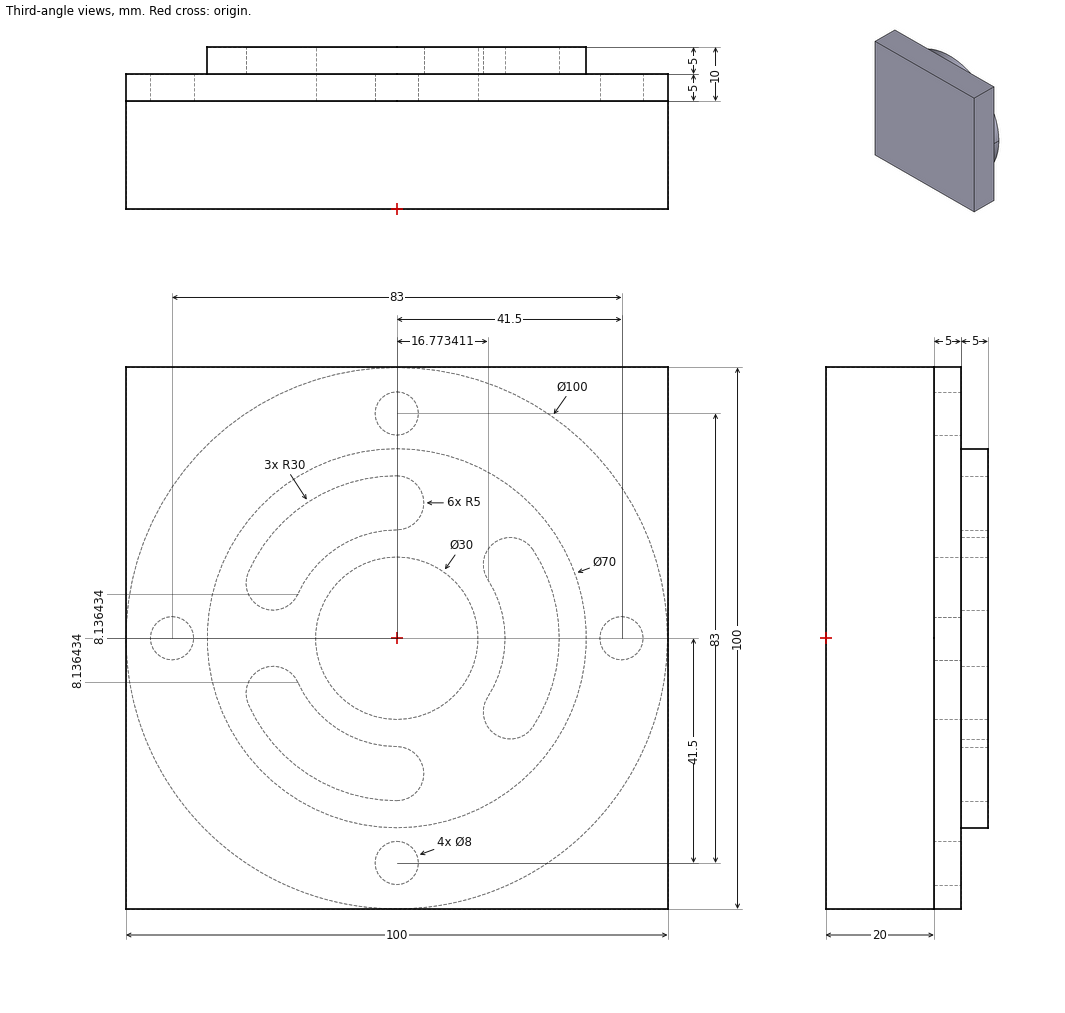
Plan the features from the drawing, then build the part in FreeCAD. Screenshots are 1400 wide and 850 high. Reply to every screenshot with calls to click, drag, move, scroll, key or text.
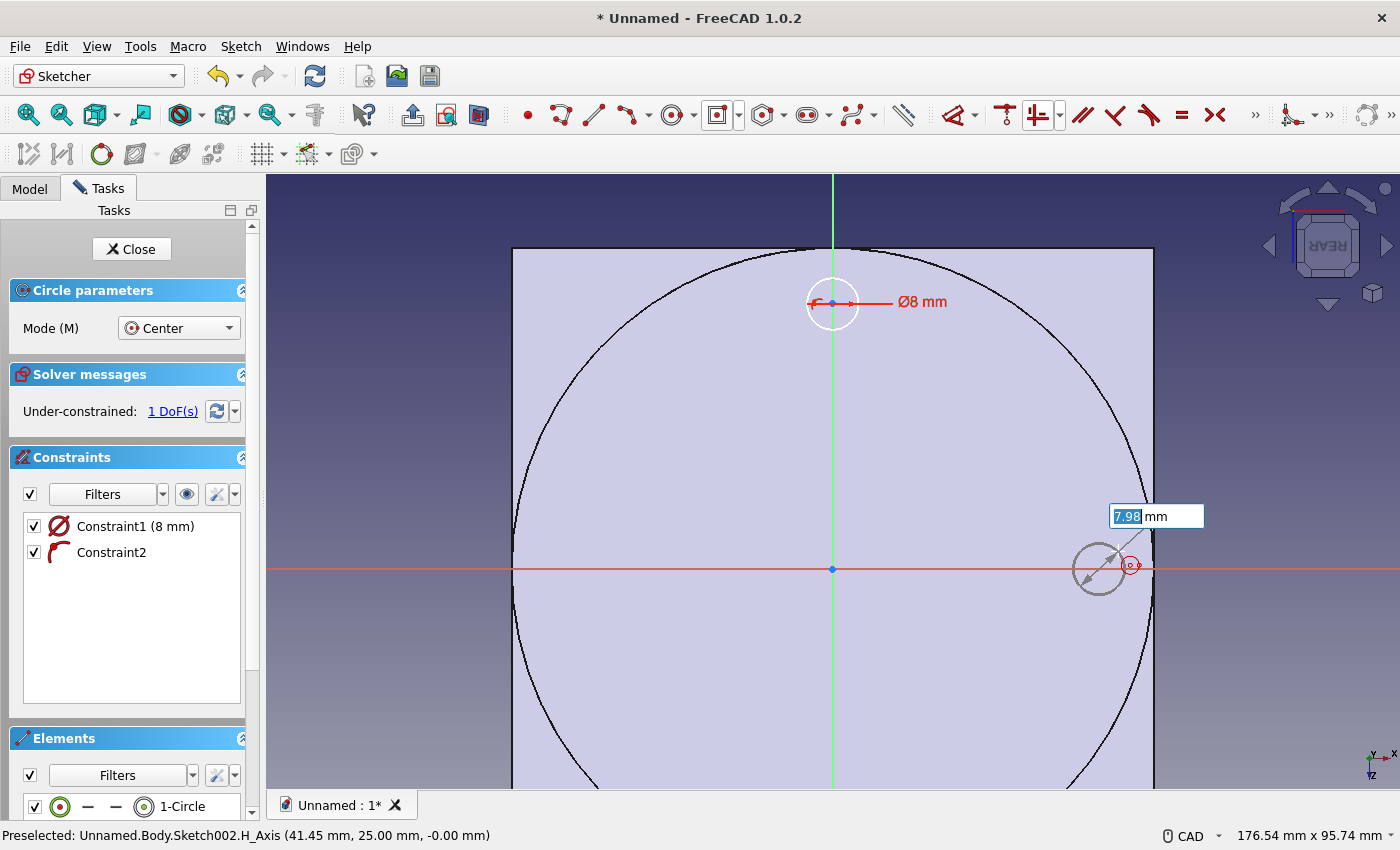
text(8)
key(Return)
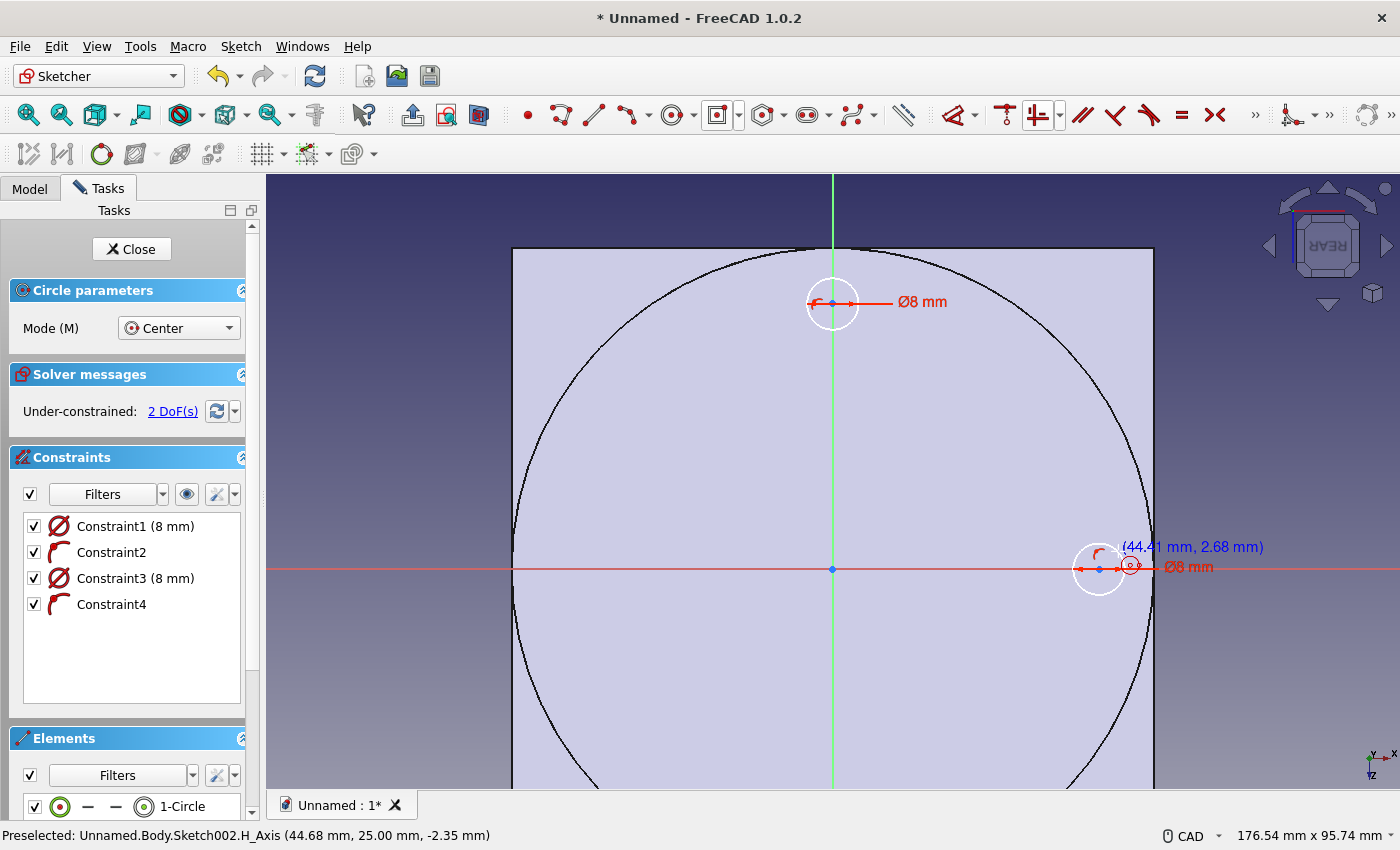
scroll(626, 303, down, 2)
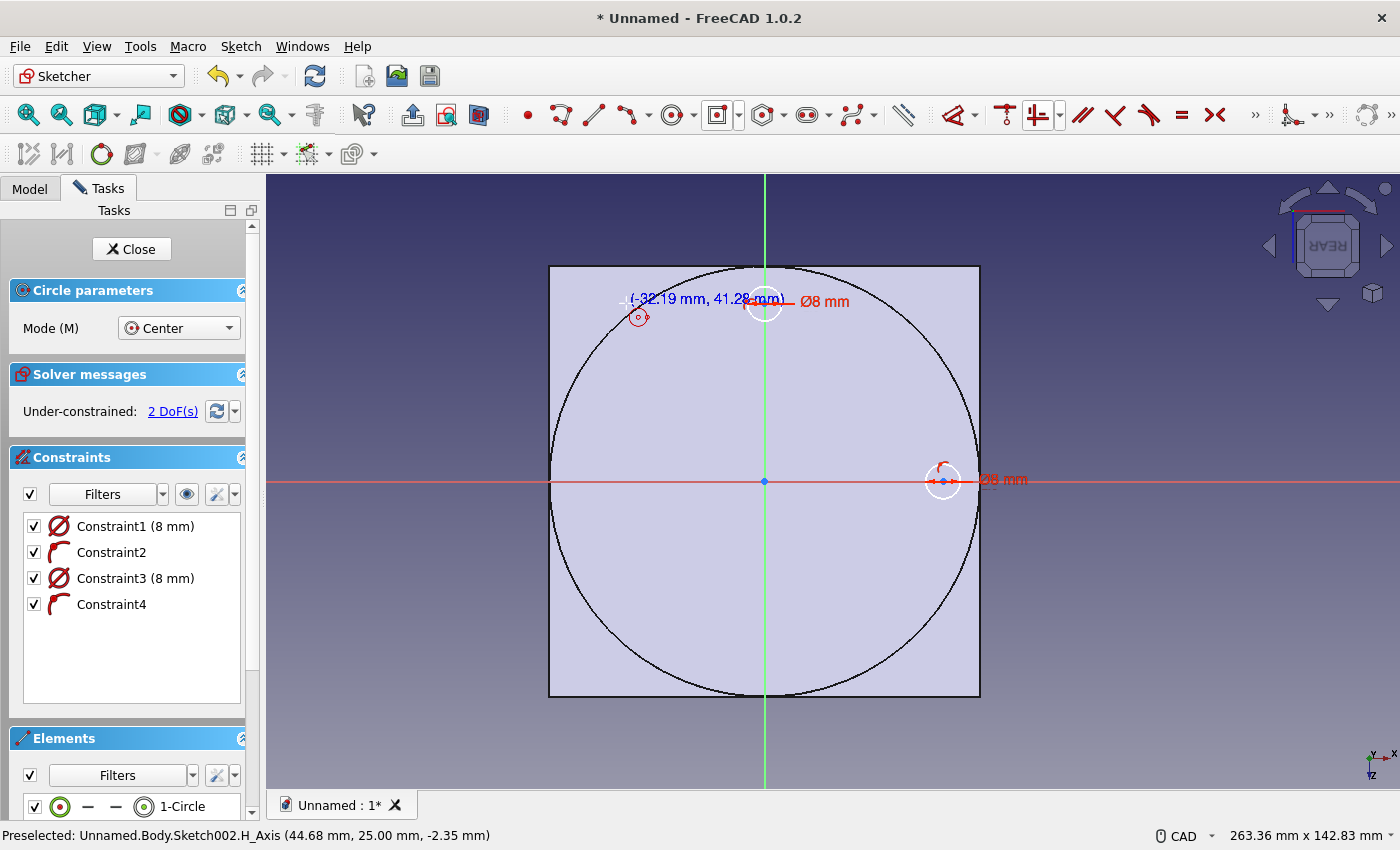
scroll(765, 660, up, 2)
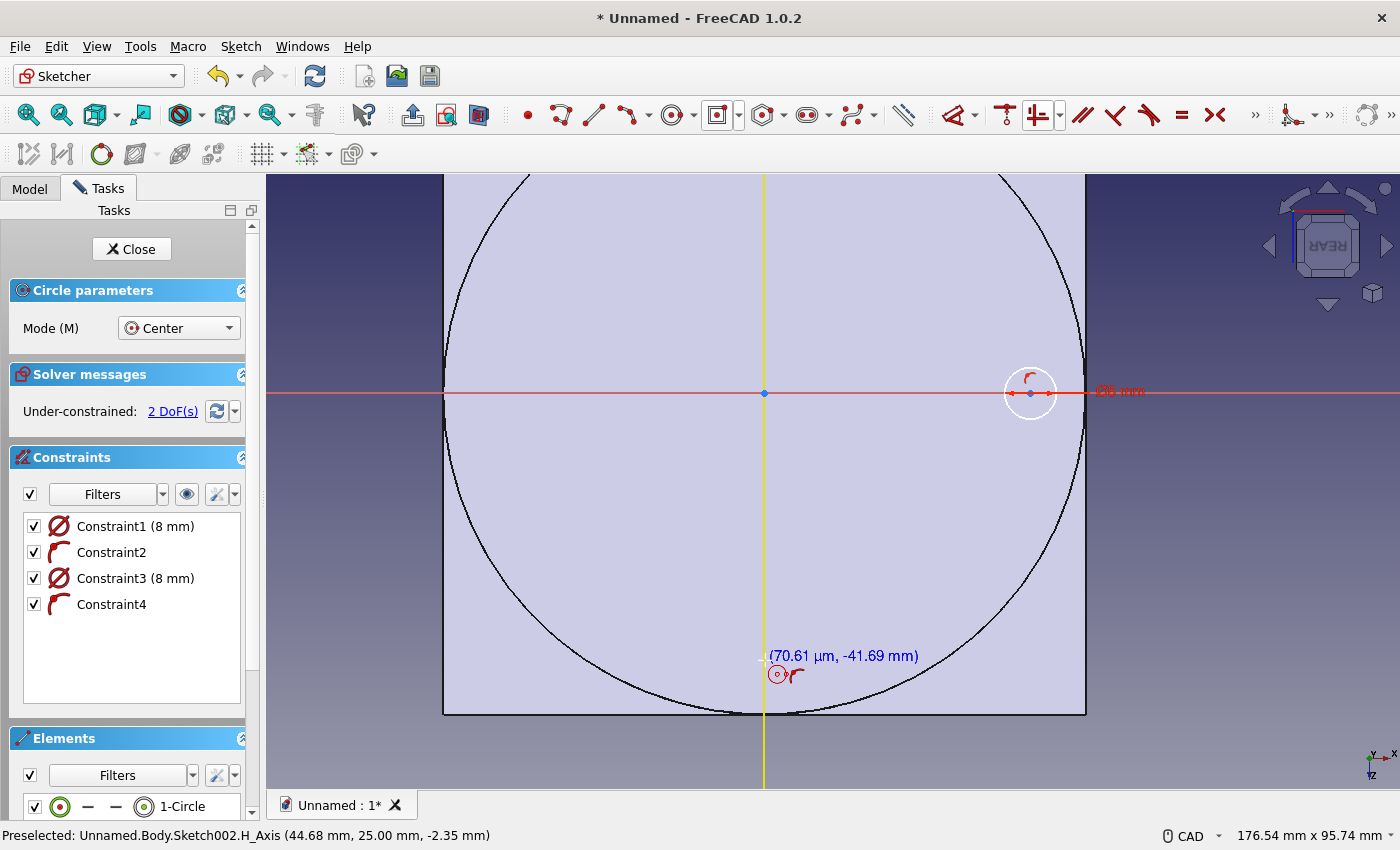
click(764, 660)
move(782, 642)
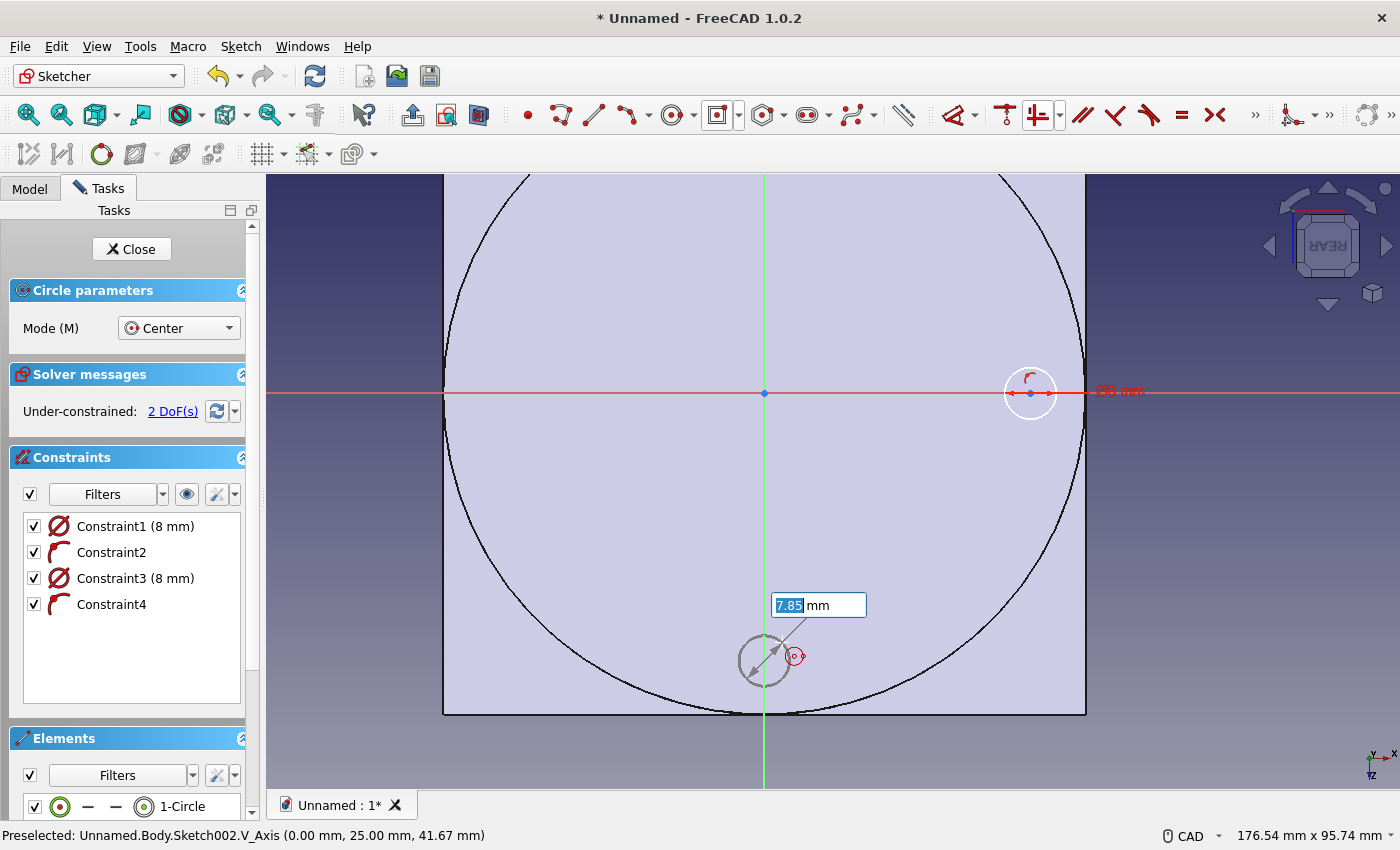
text(8)
key(Return)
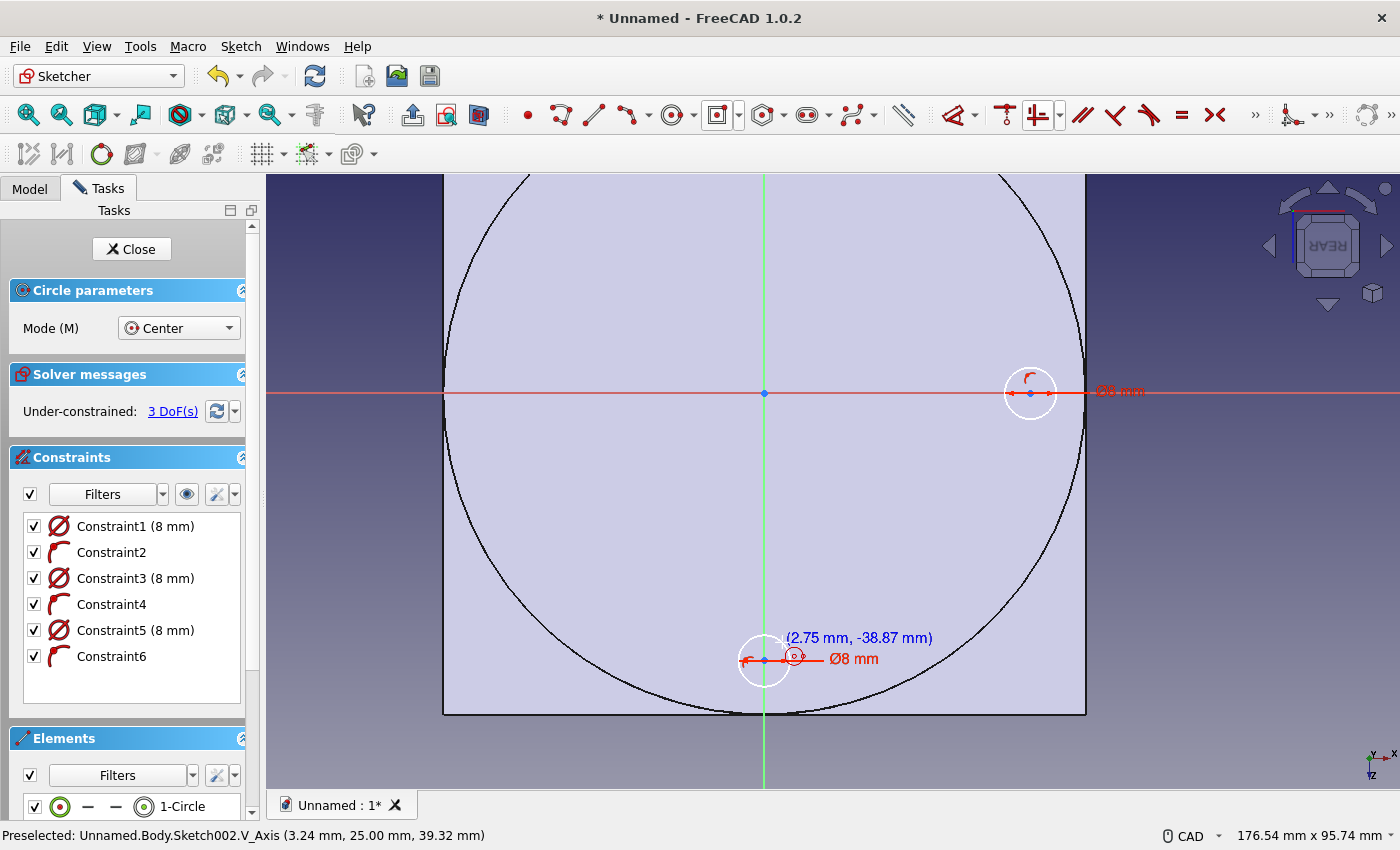
click(498, 393)
move(516, 375)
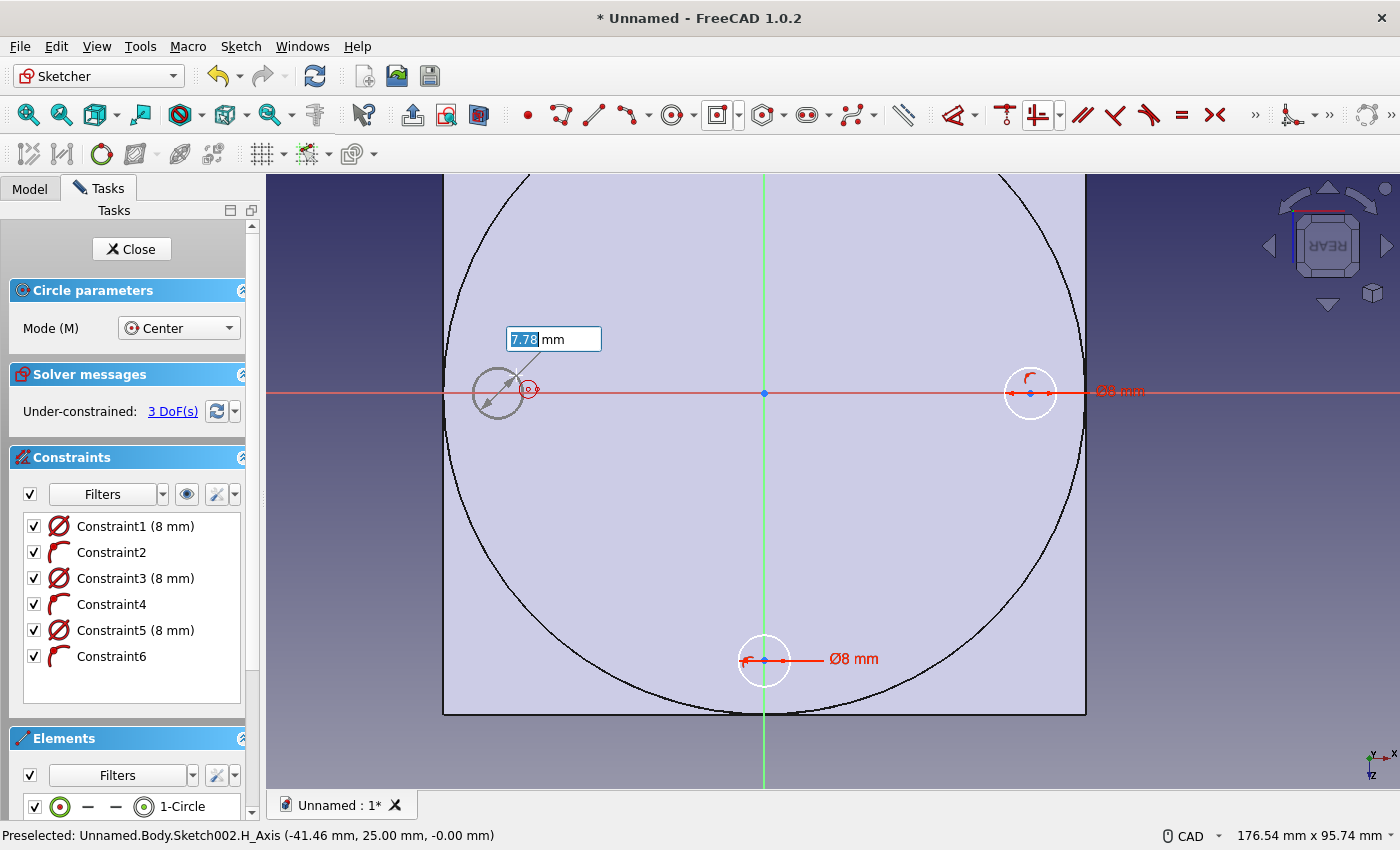
text(8)
key(Return)
key(Escape)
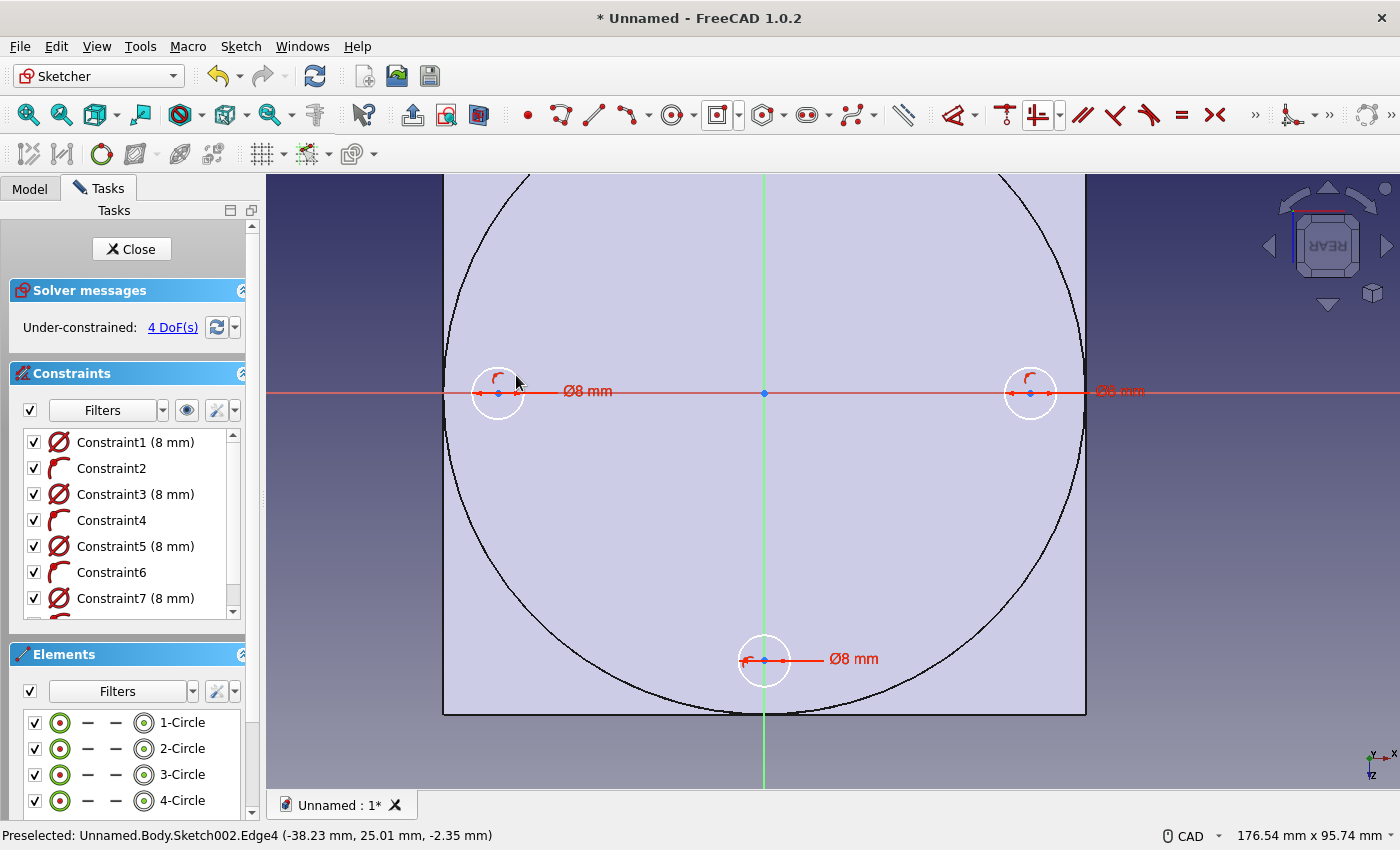
scroll(765, 661, down, 2)